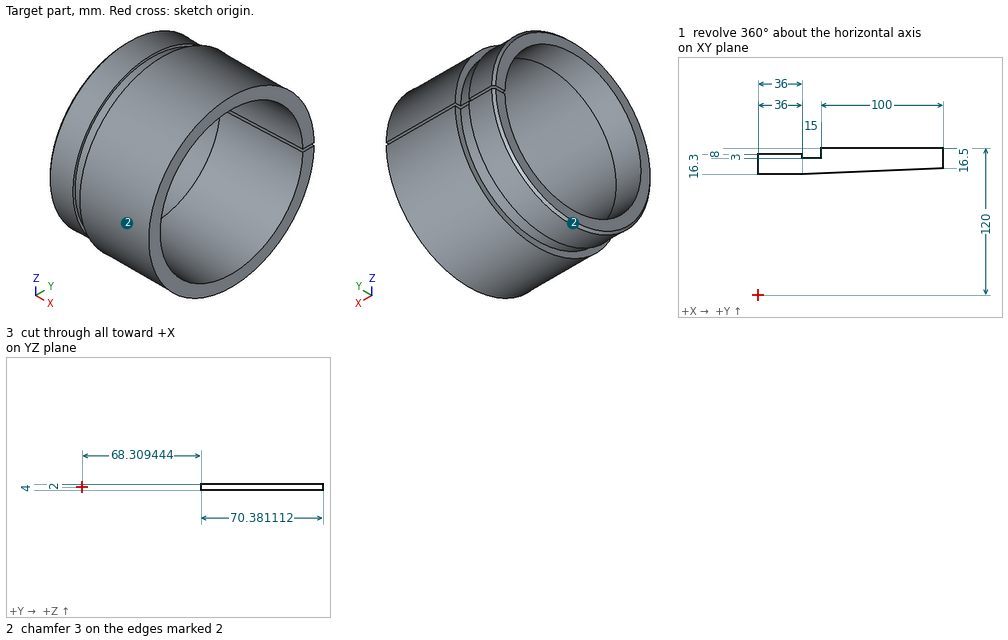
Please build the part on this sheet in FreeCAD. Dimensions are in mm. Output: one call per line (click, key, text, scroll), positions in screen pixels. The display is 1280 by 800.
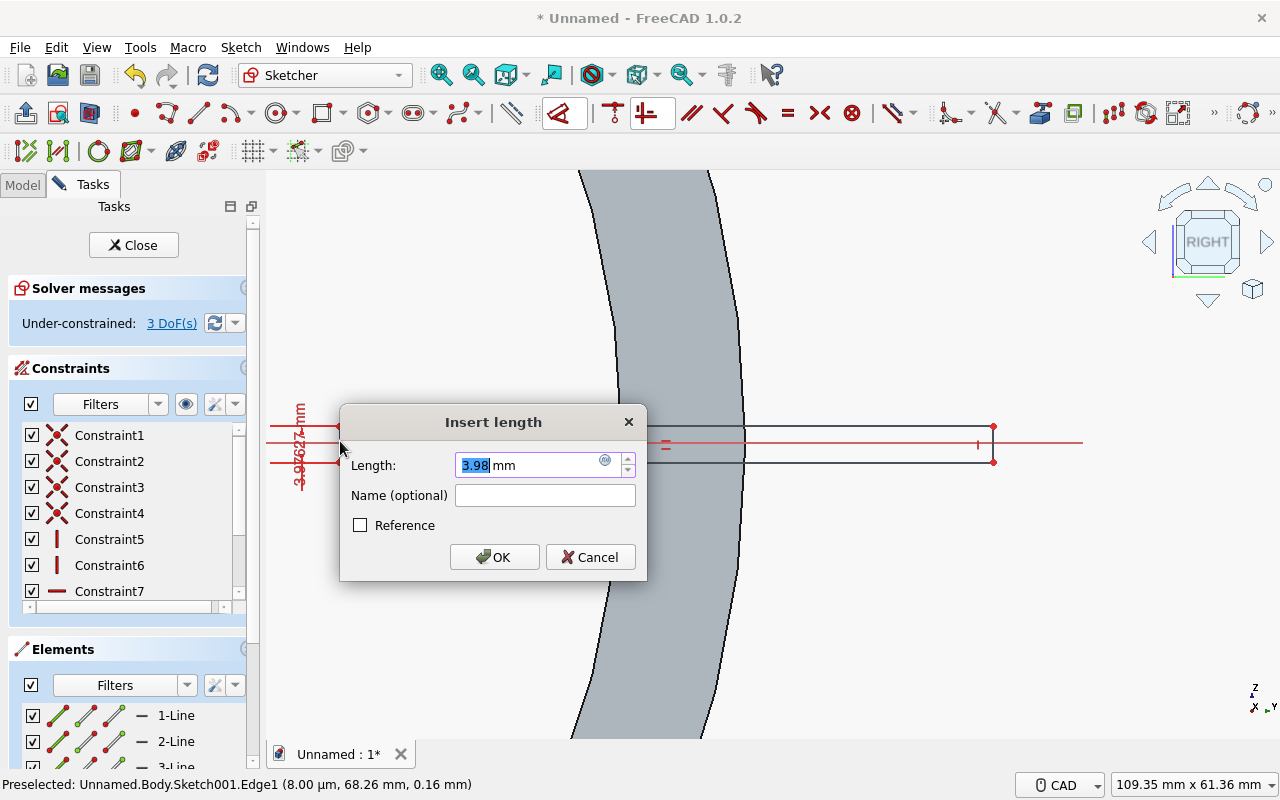
text(4)
key(Return)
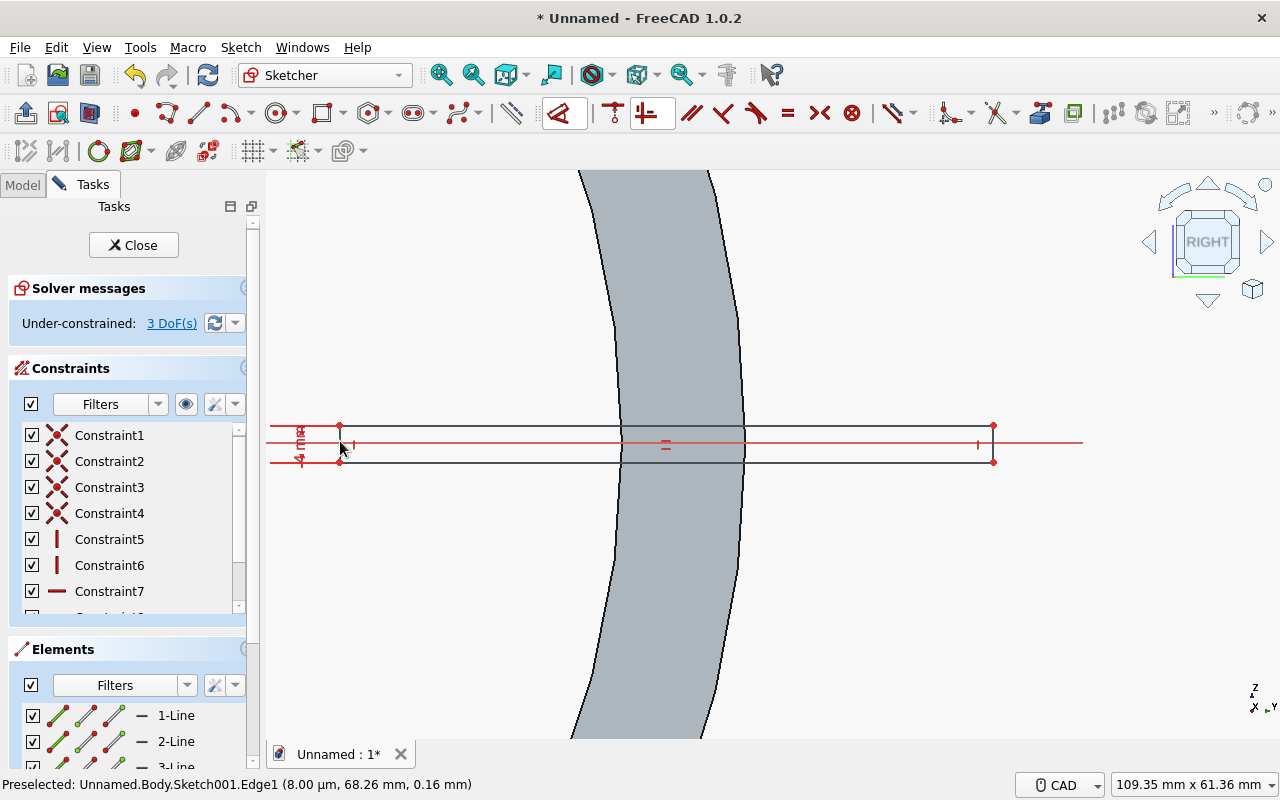
scroll(340, 426, up, 4)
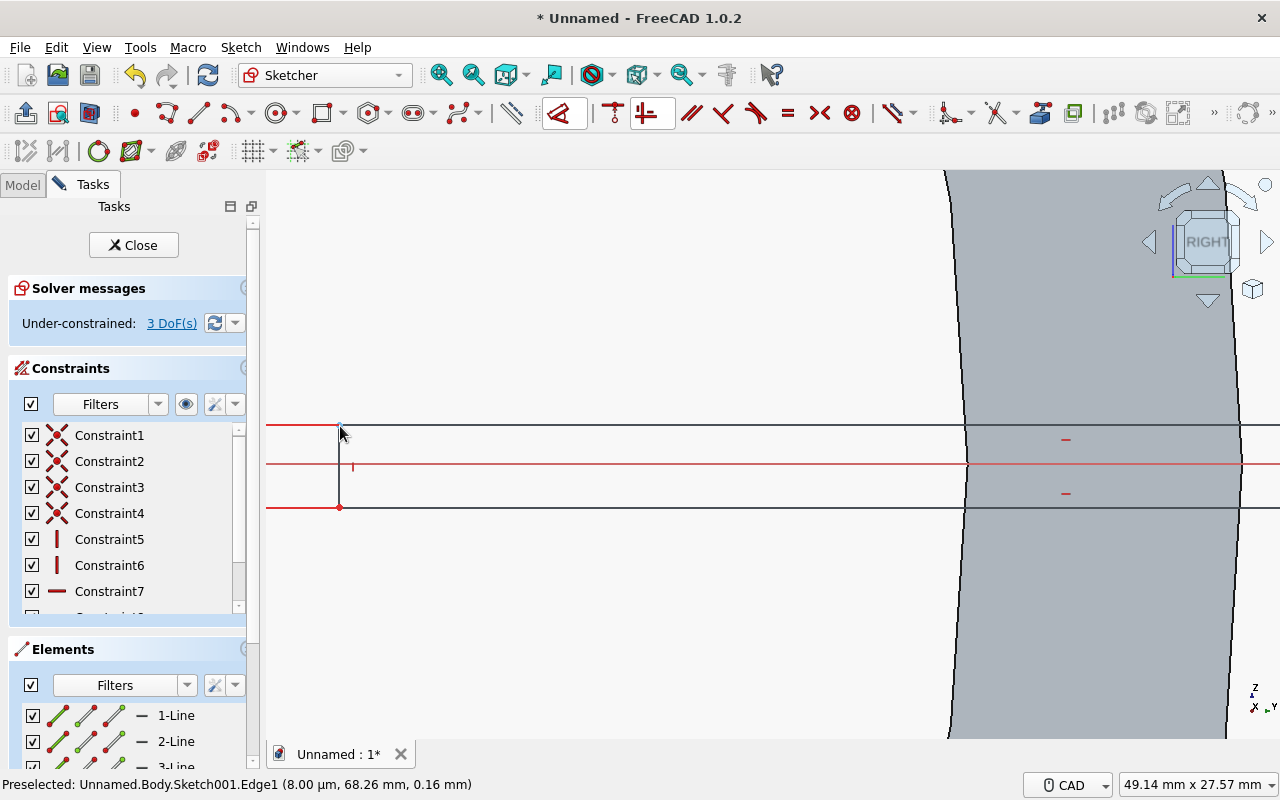
click(339, 425)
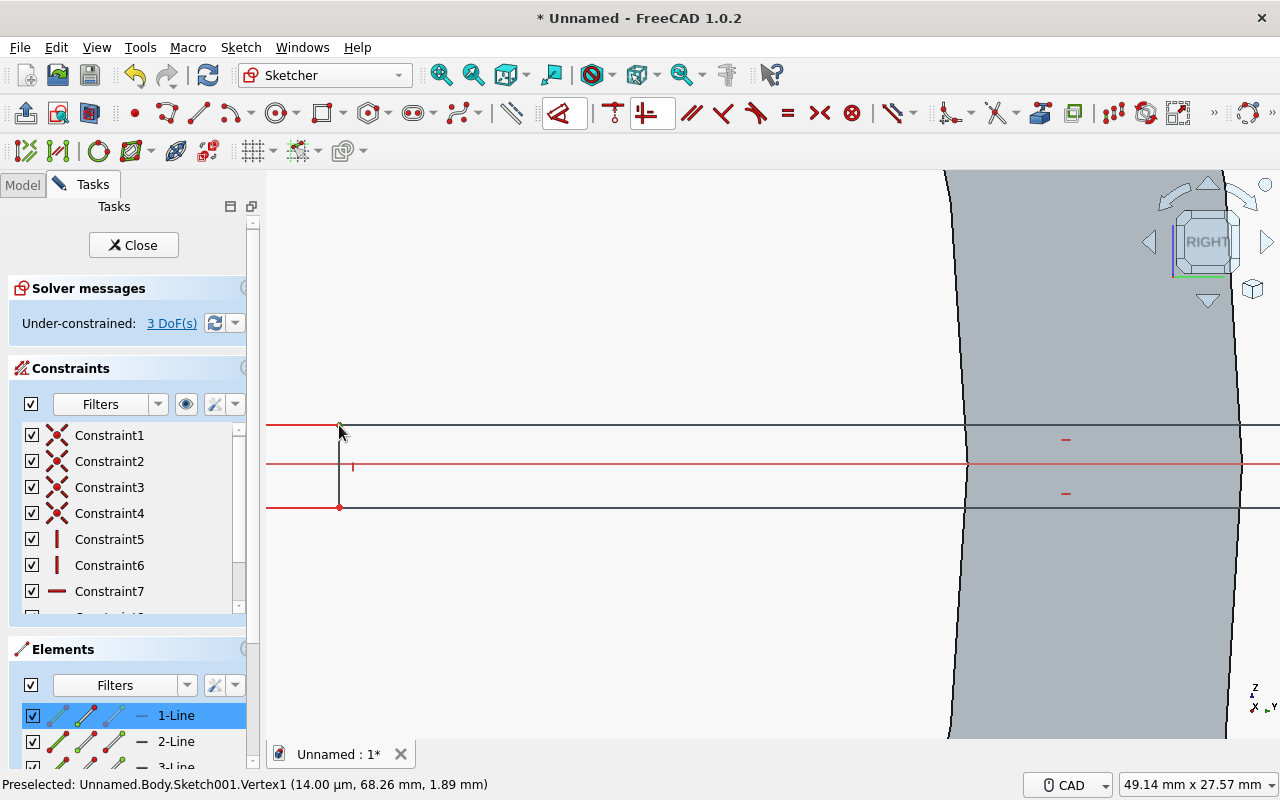
click(582, 114)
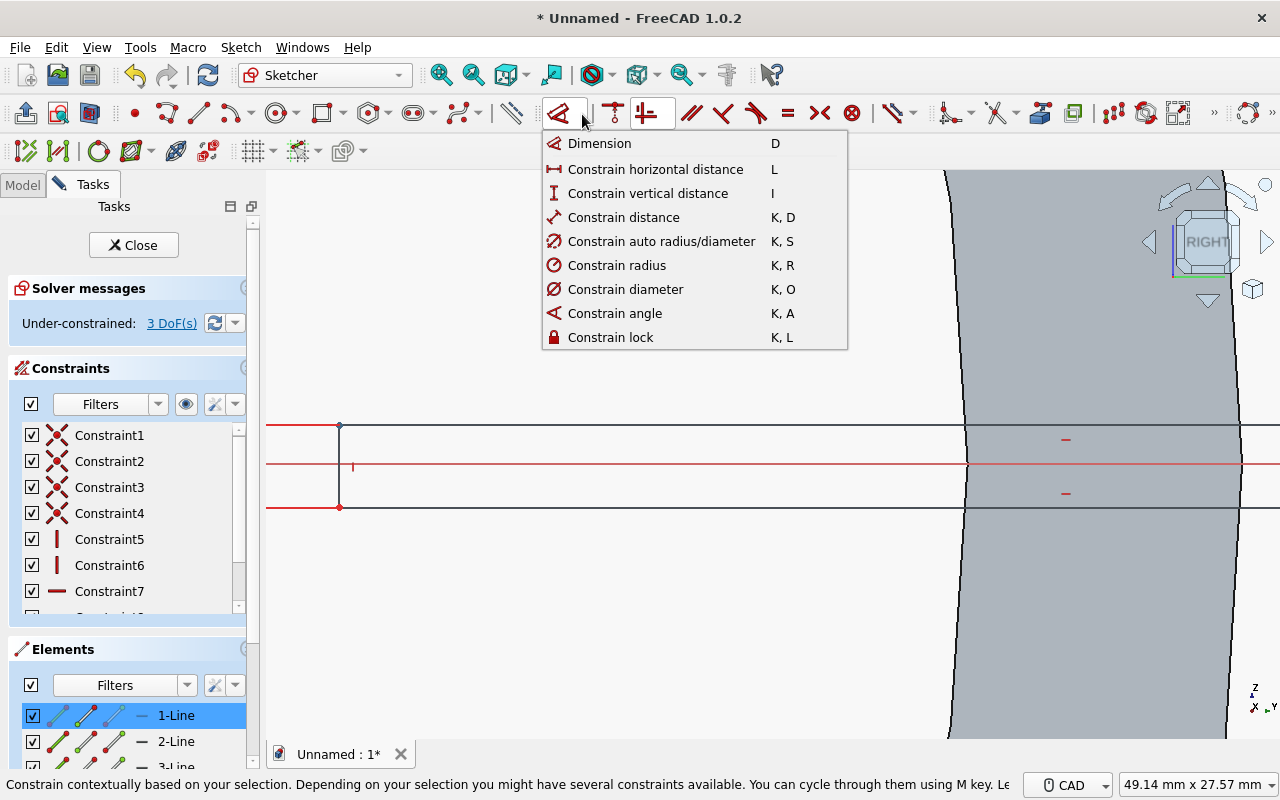
click(695, 193)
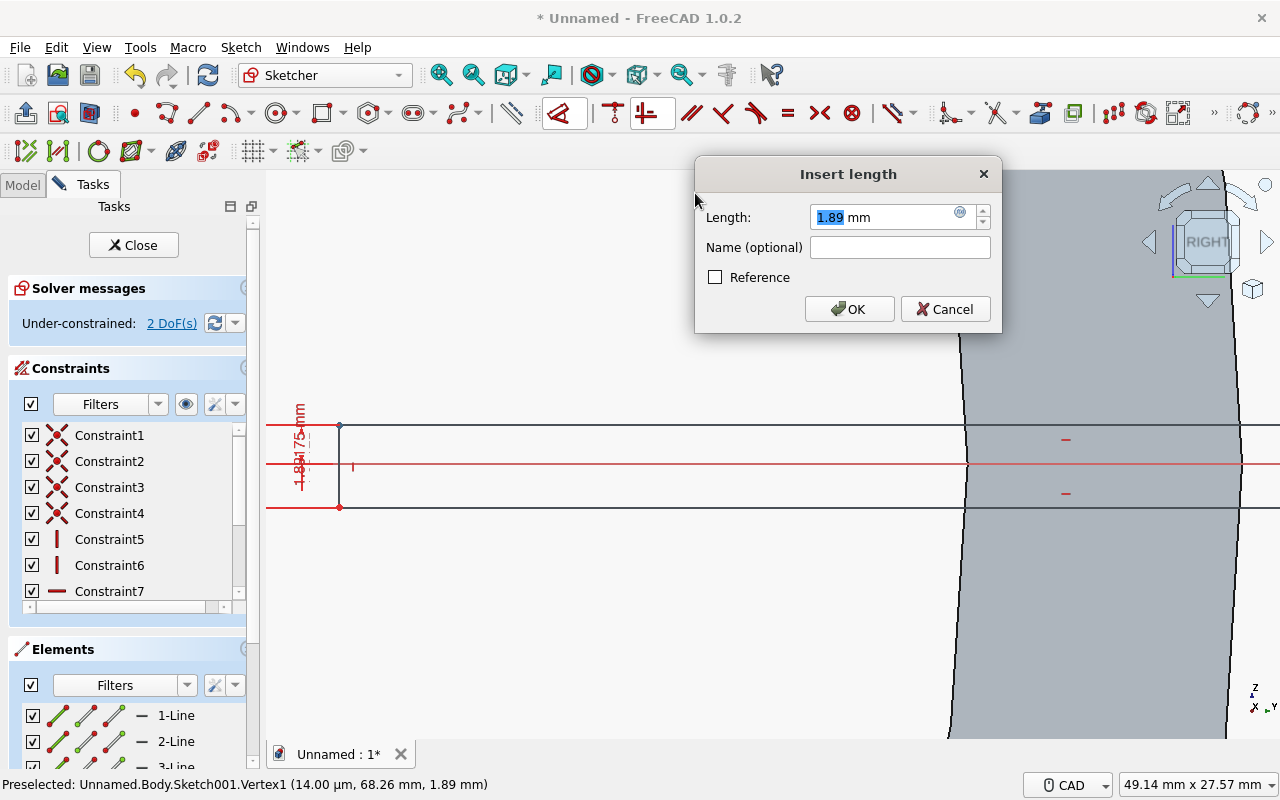
text(2)
key(Return)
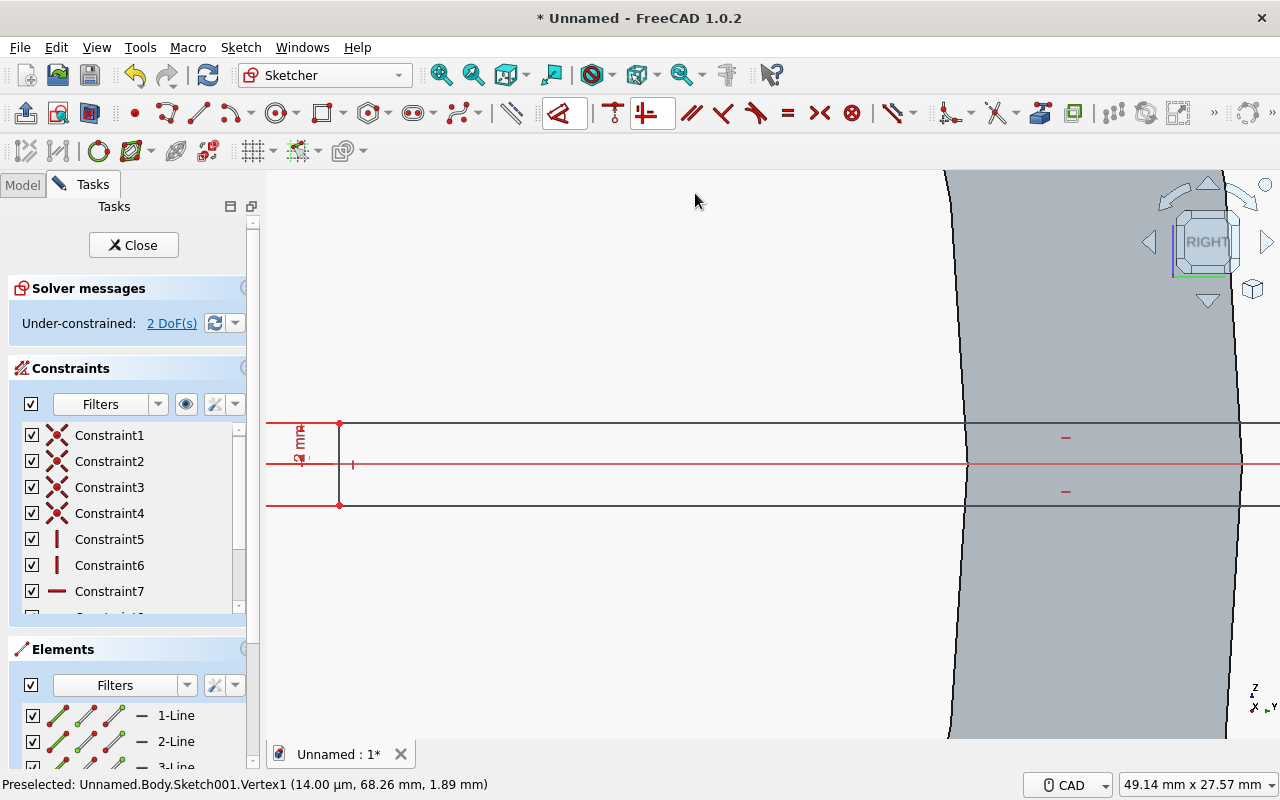
scroll(791, 452, down, 8)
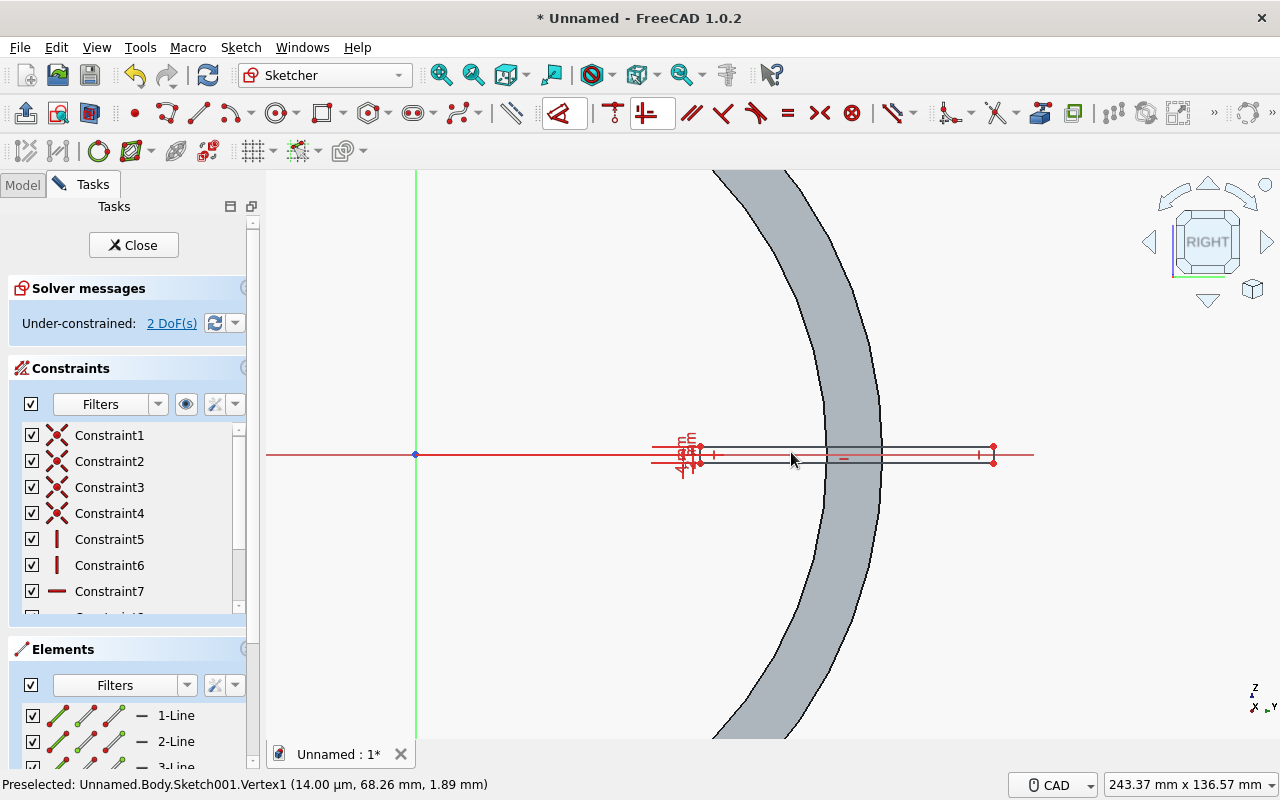
scroll(788, 463, up, 3)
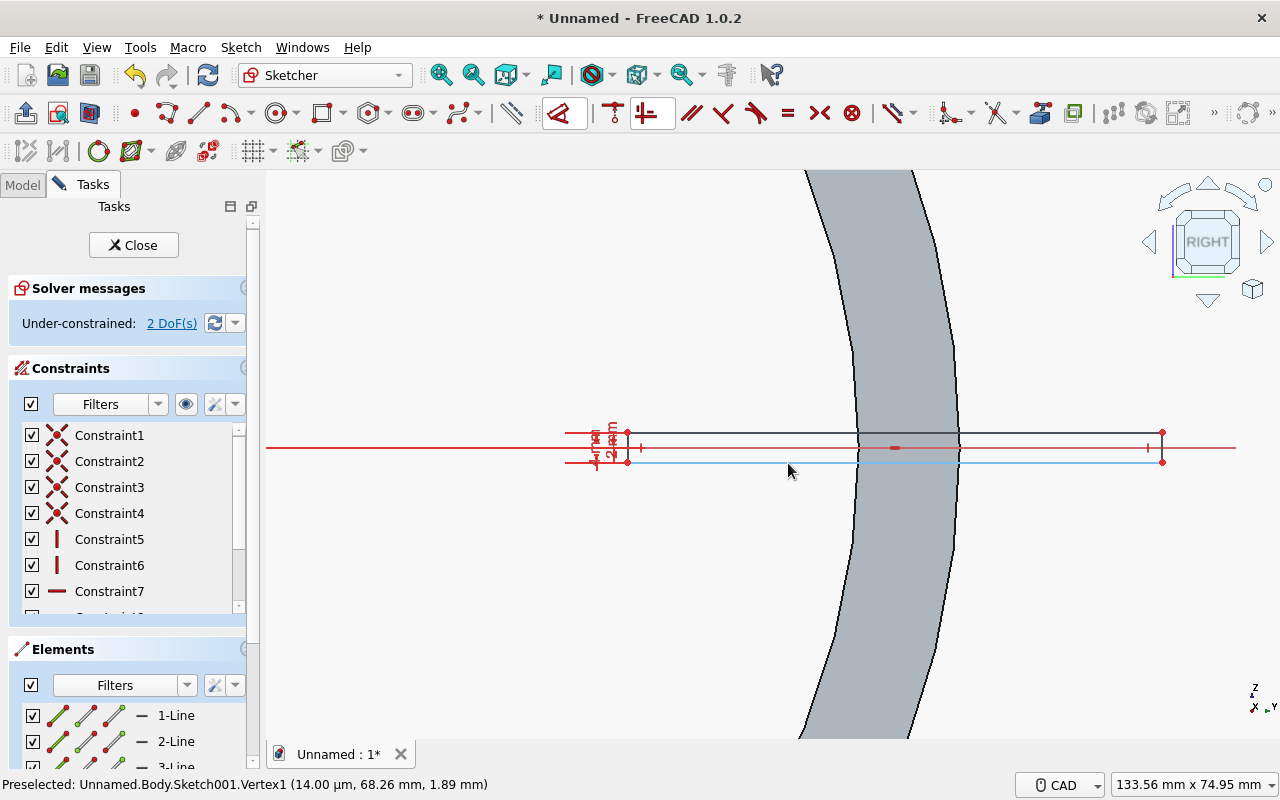
click(788, 463)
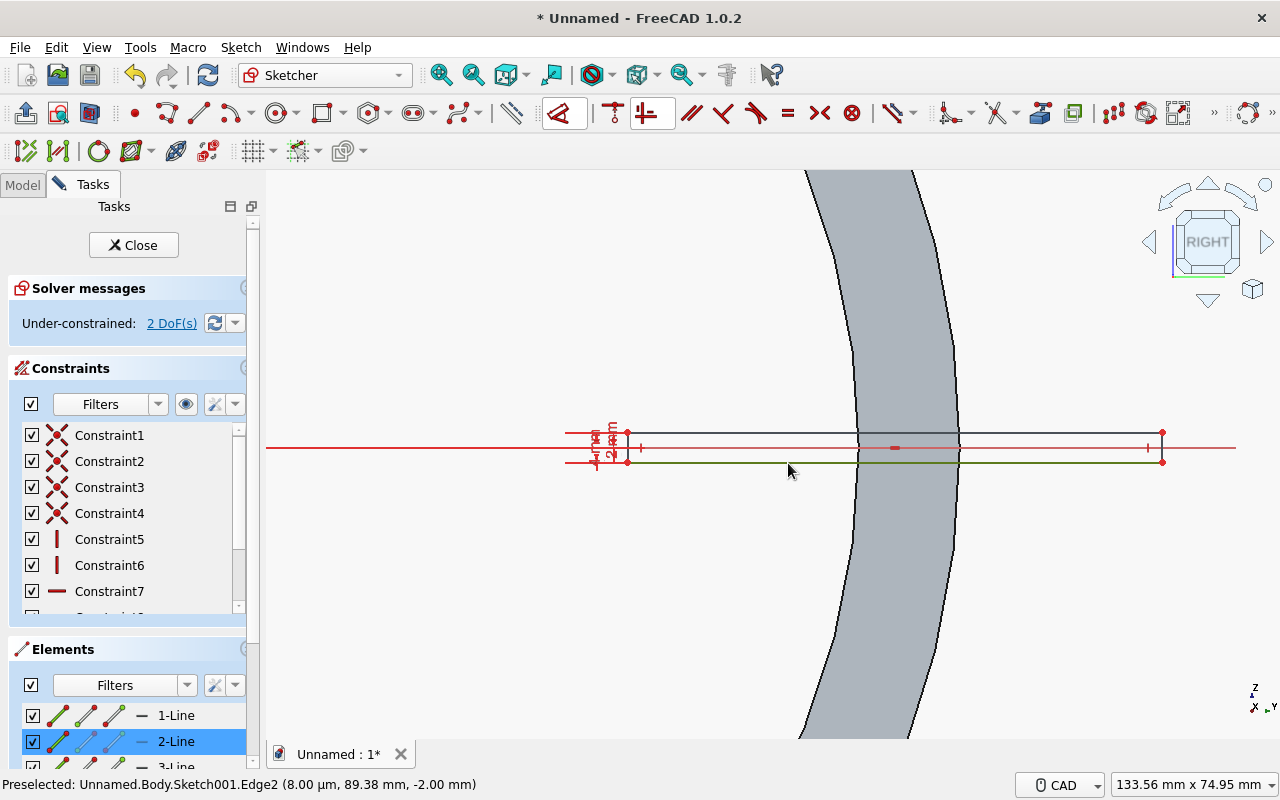
key(l)